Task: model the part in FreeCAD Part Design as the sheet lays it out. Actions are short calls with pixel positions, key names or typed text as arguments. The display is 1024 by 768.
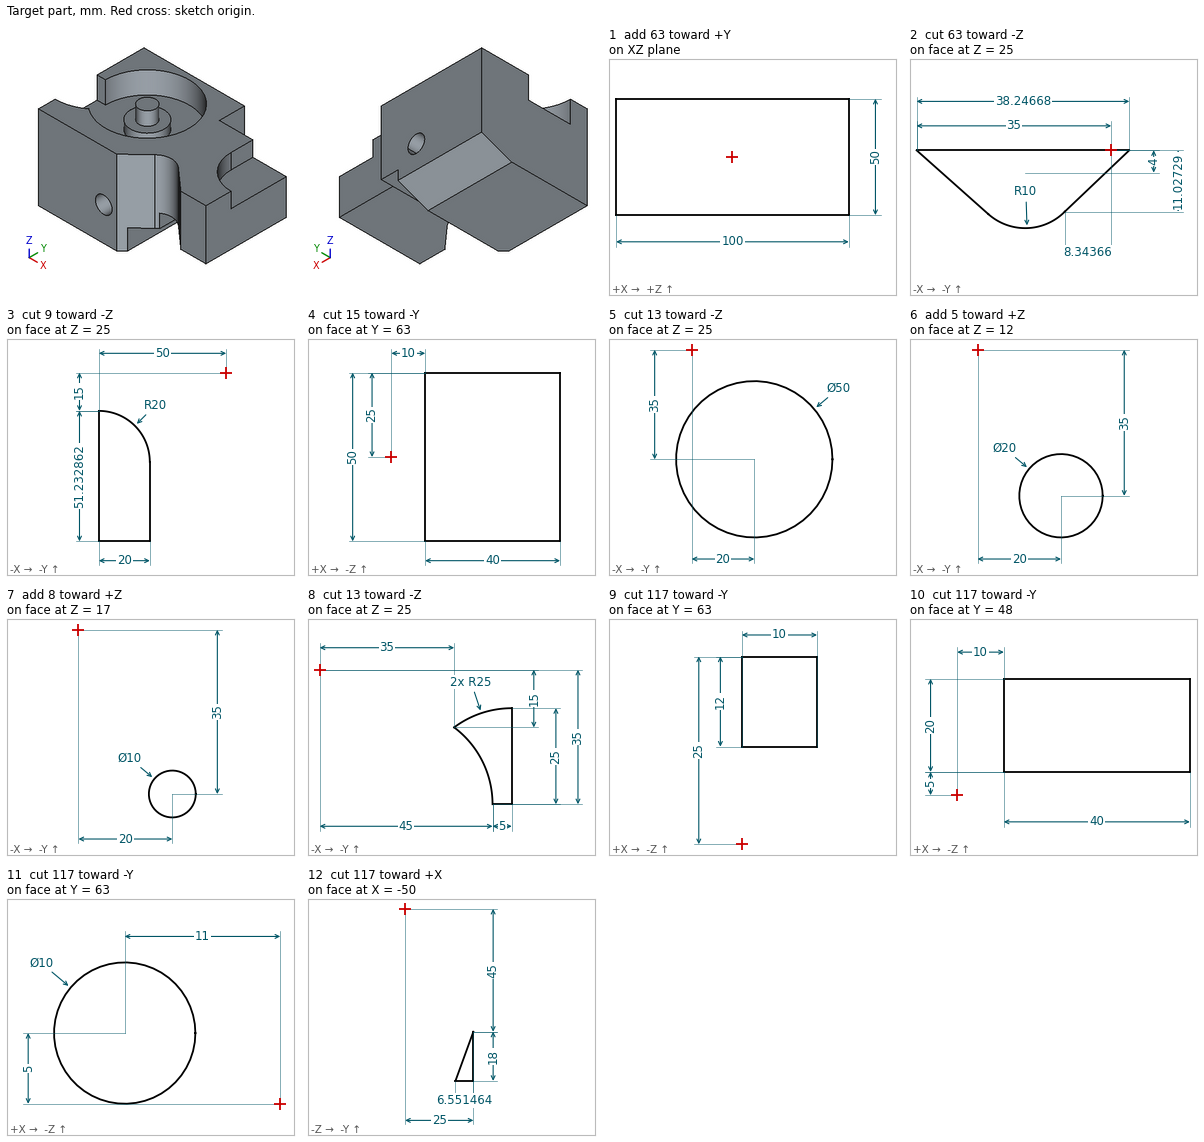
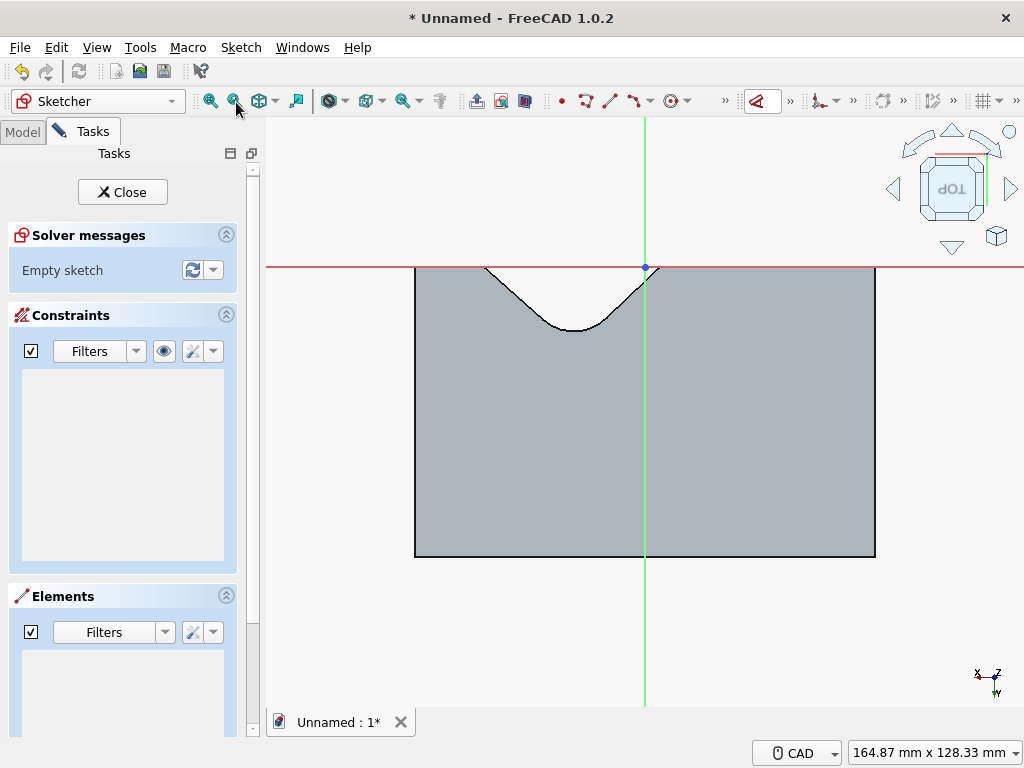
click(586, 102)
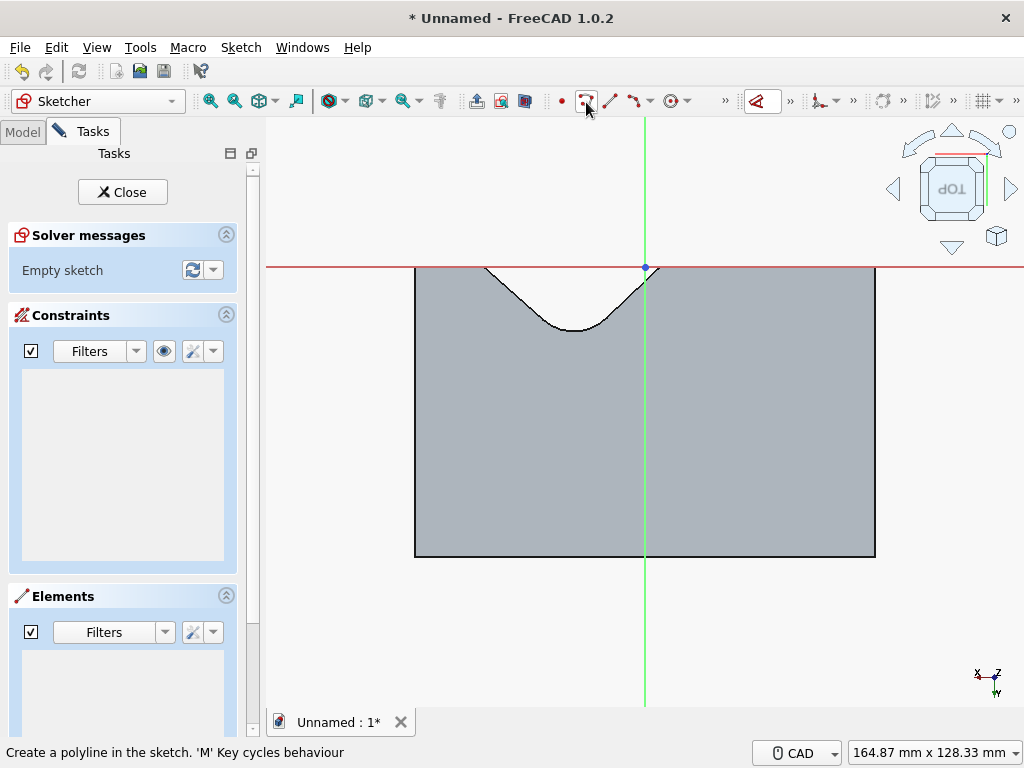
click(415, 336)
click(415, 572)
click(507, 572)
click(507, 428)
right_click(507, 428)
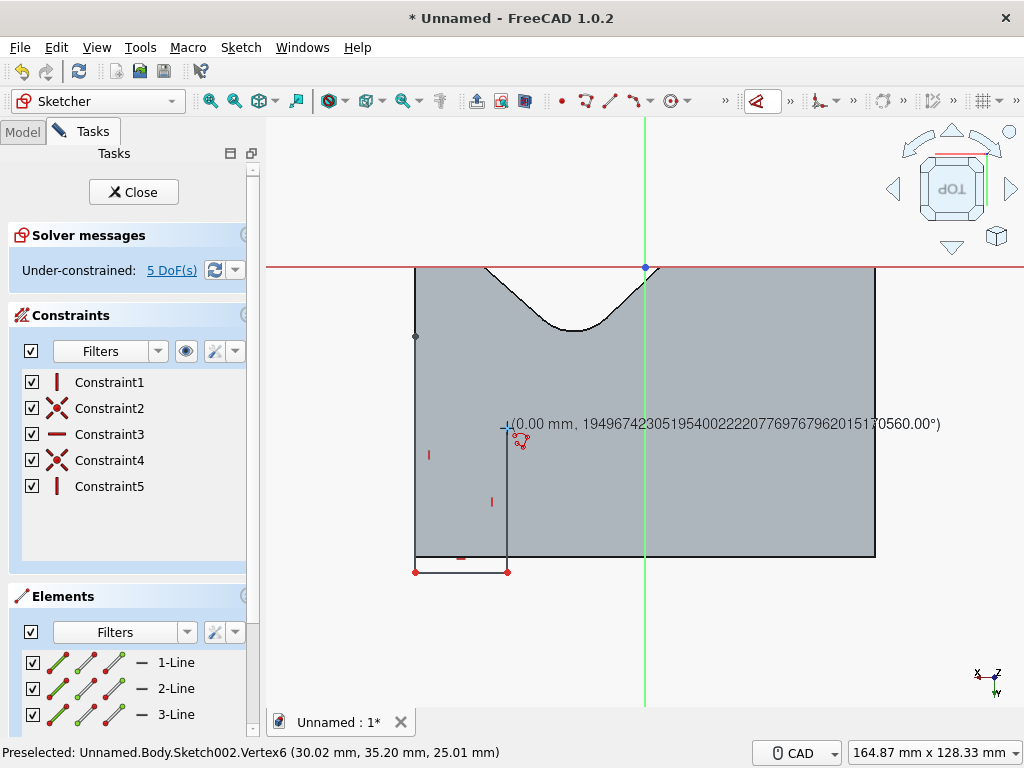
click(634, 102)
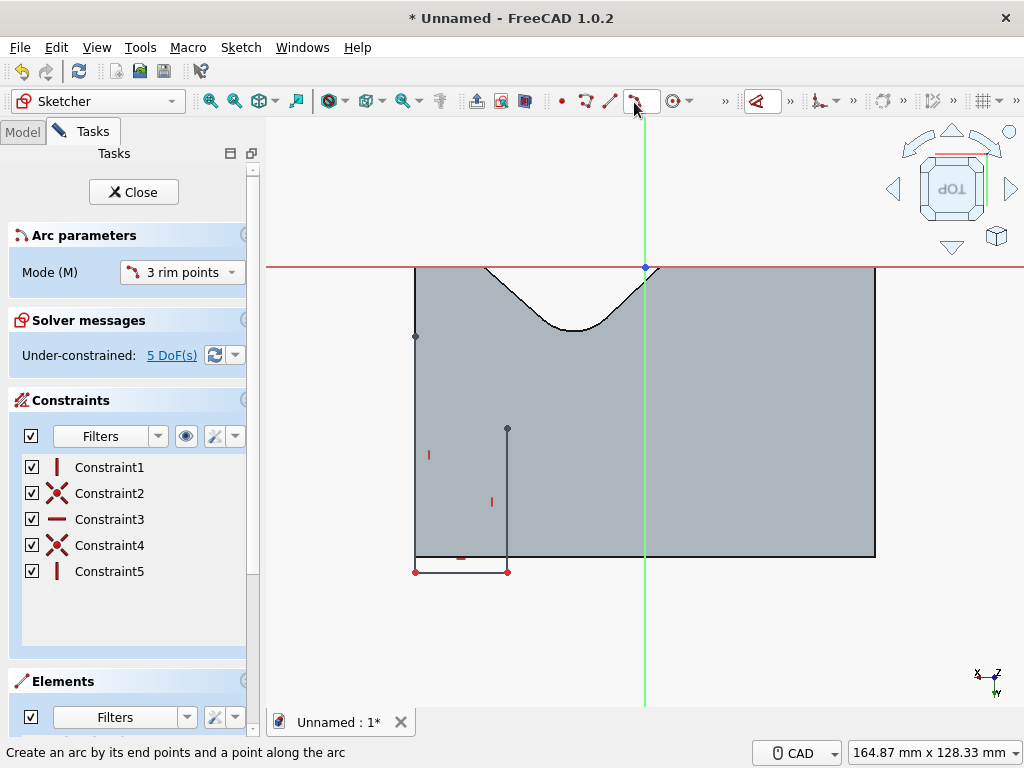
click(507, 429)
click(415, 337)
click(480, 363)
key(Escape)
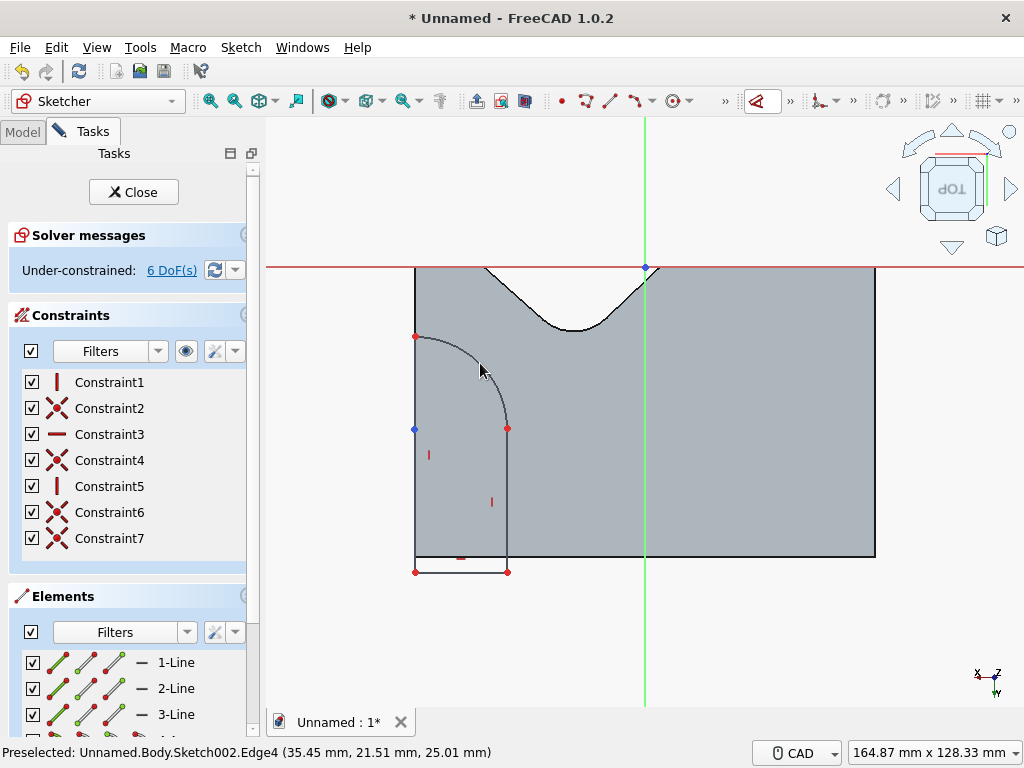
click(507, 530)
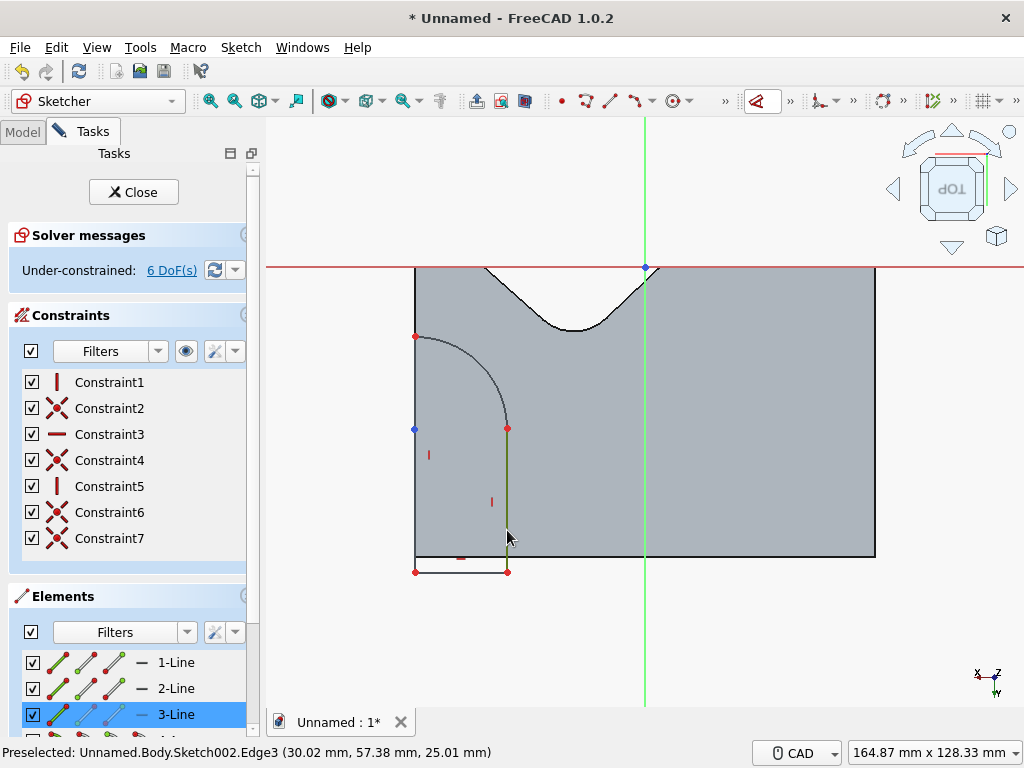
click(497, 387)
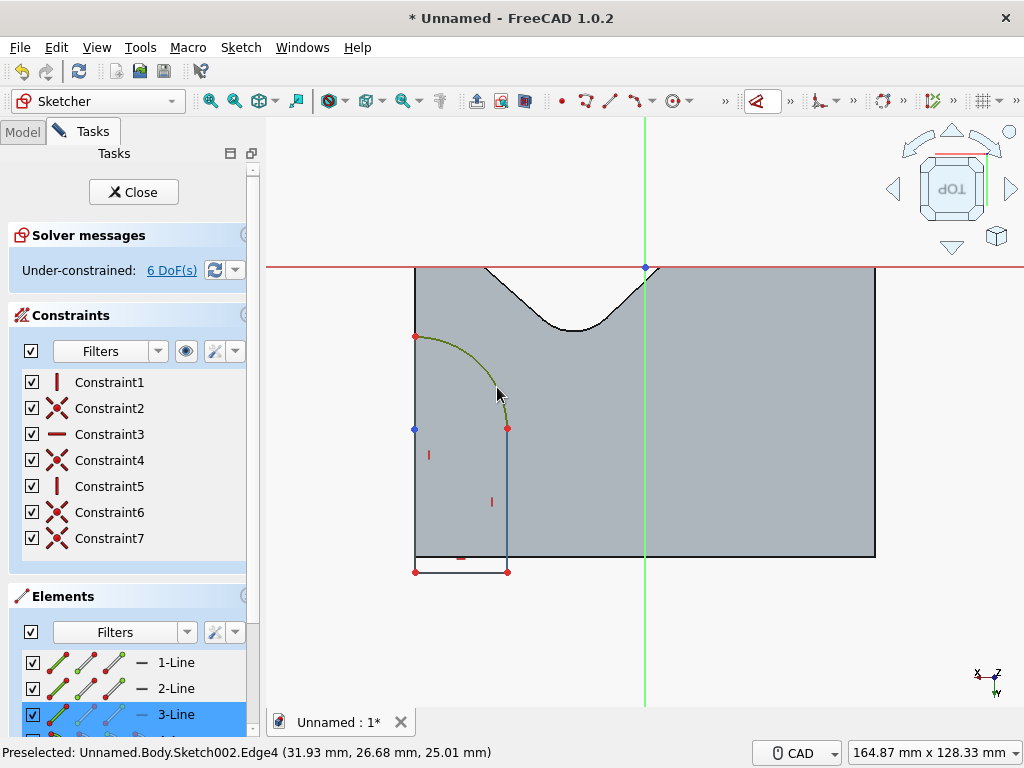
key(t)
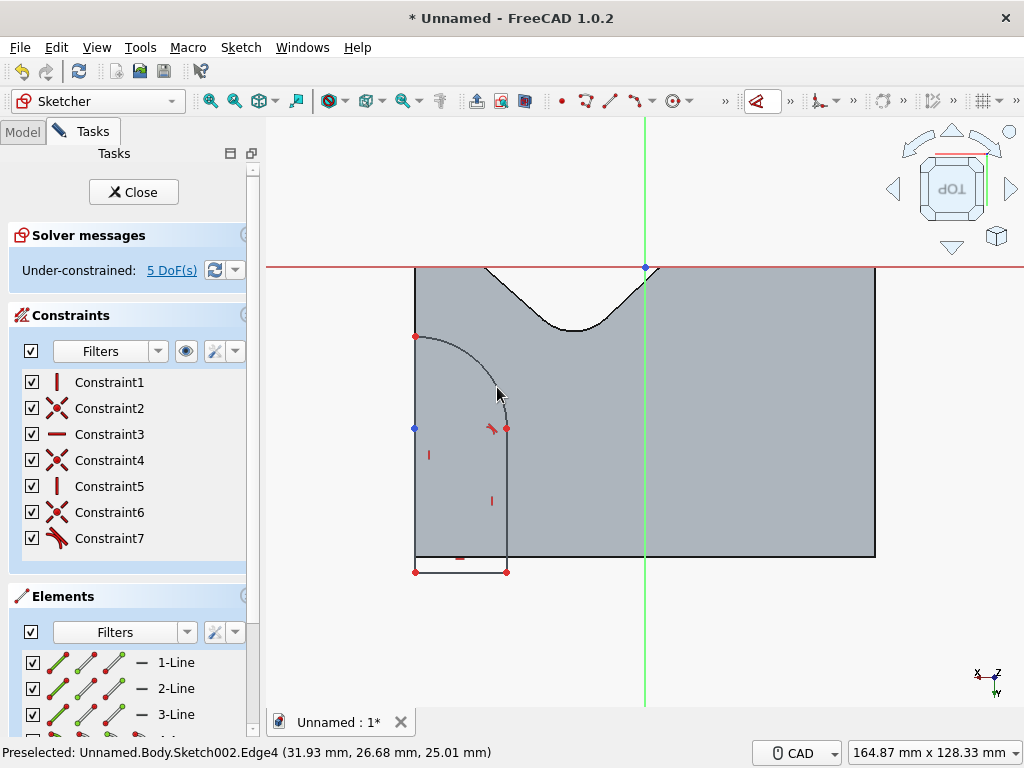
click(497, 387)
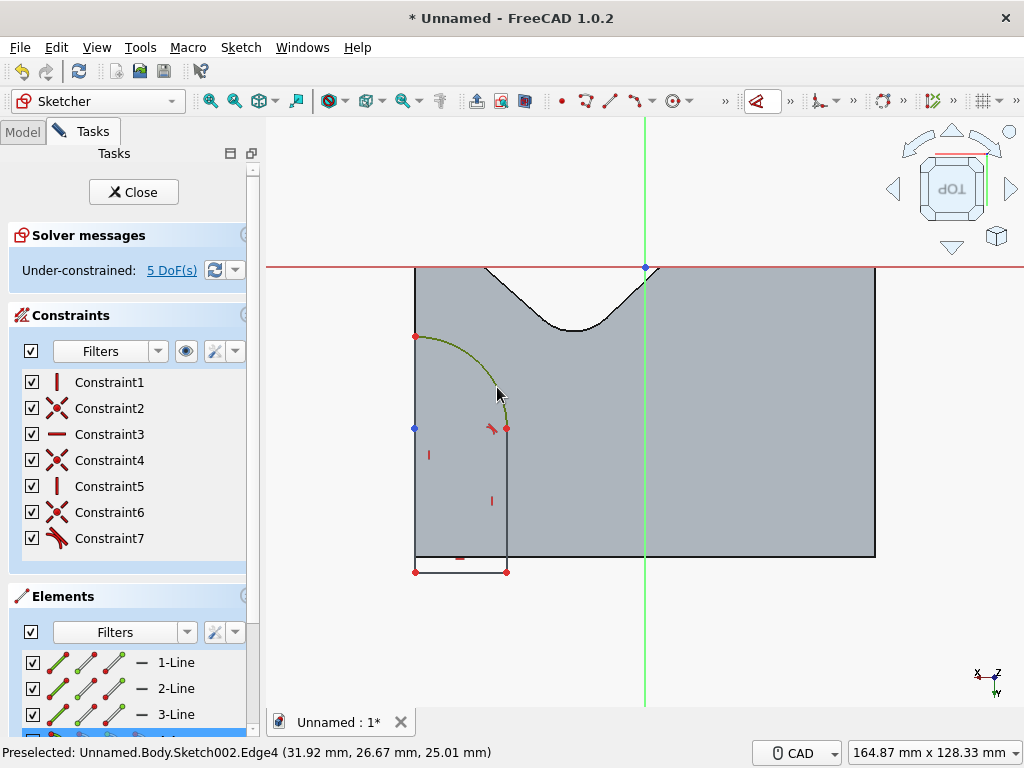
key(k)
key(r)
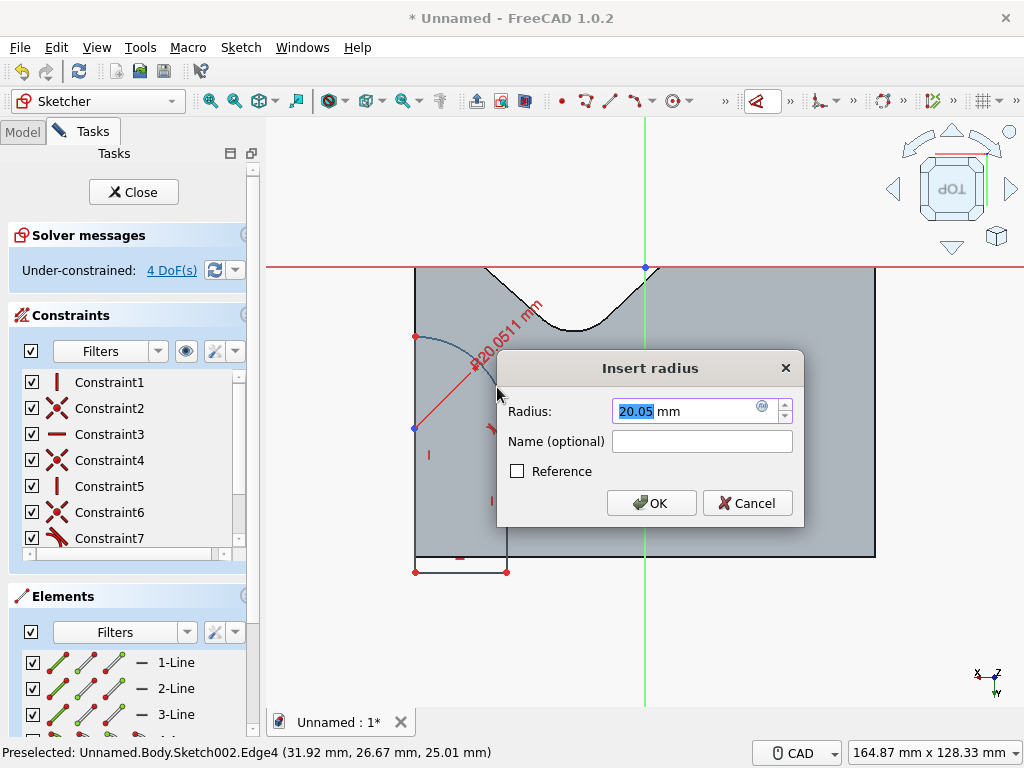
text(20)
key(Return)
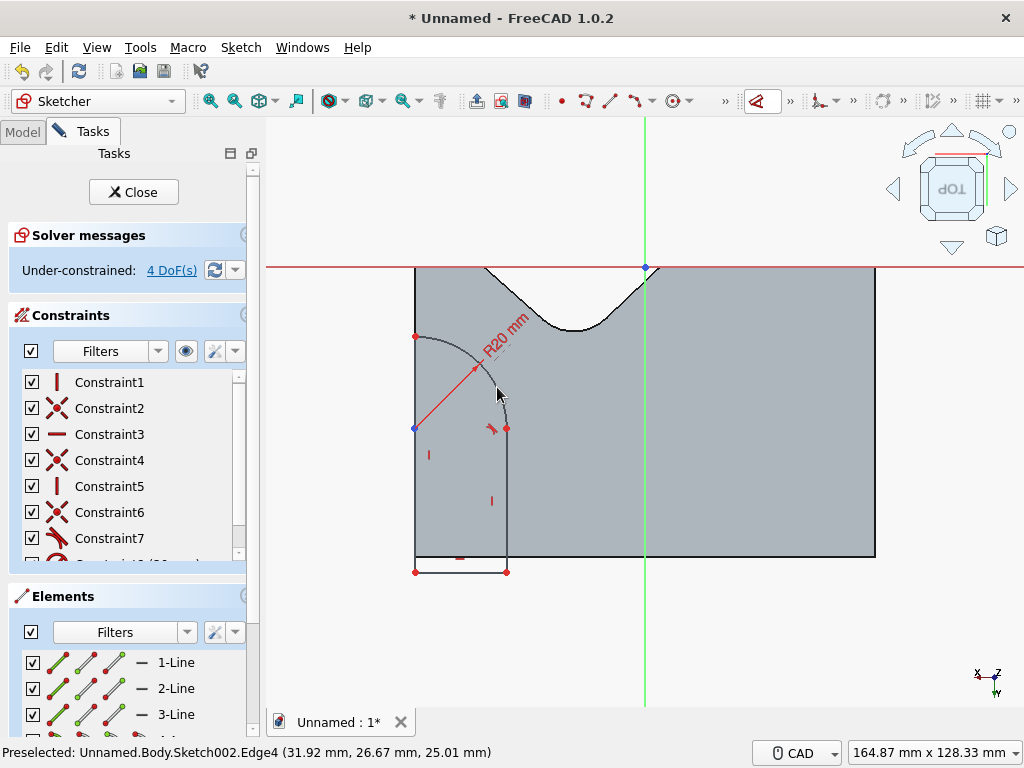
click(443, 573)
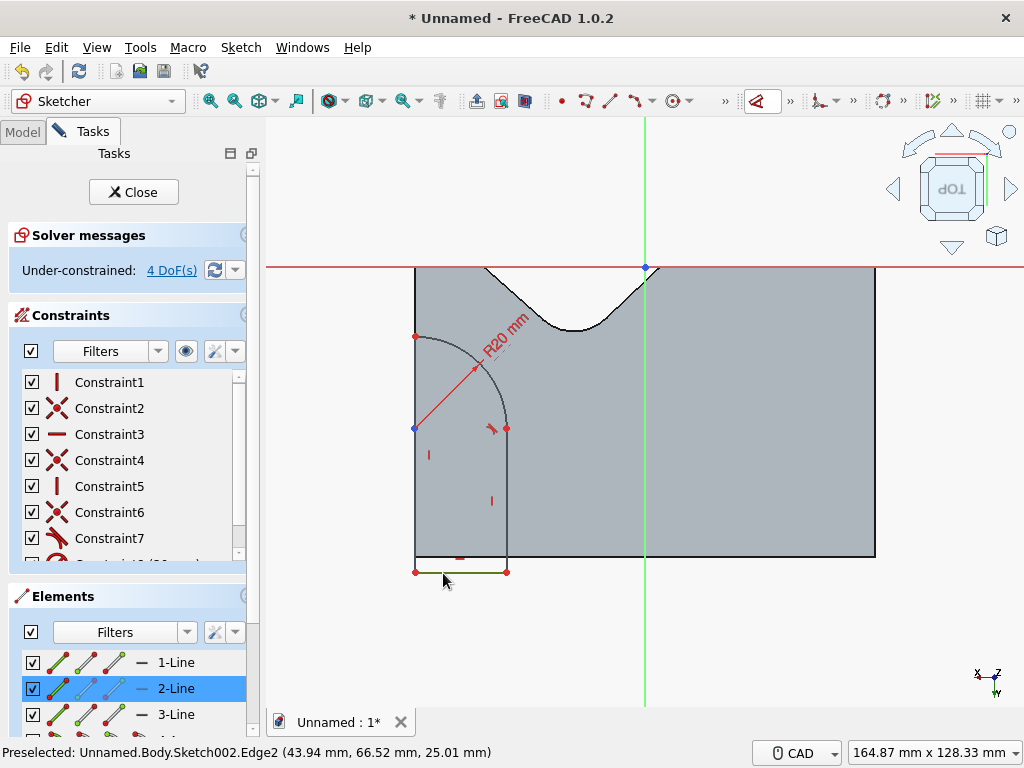
click(776, 102)